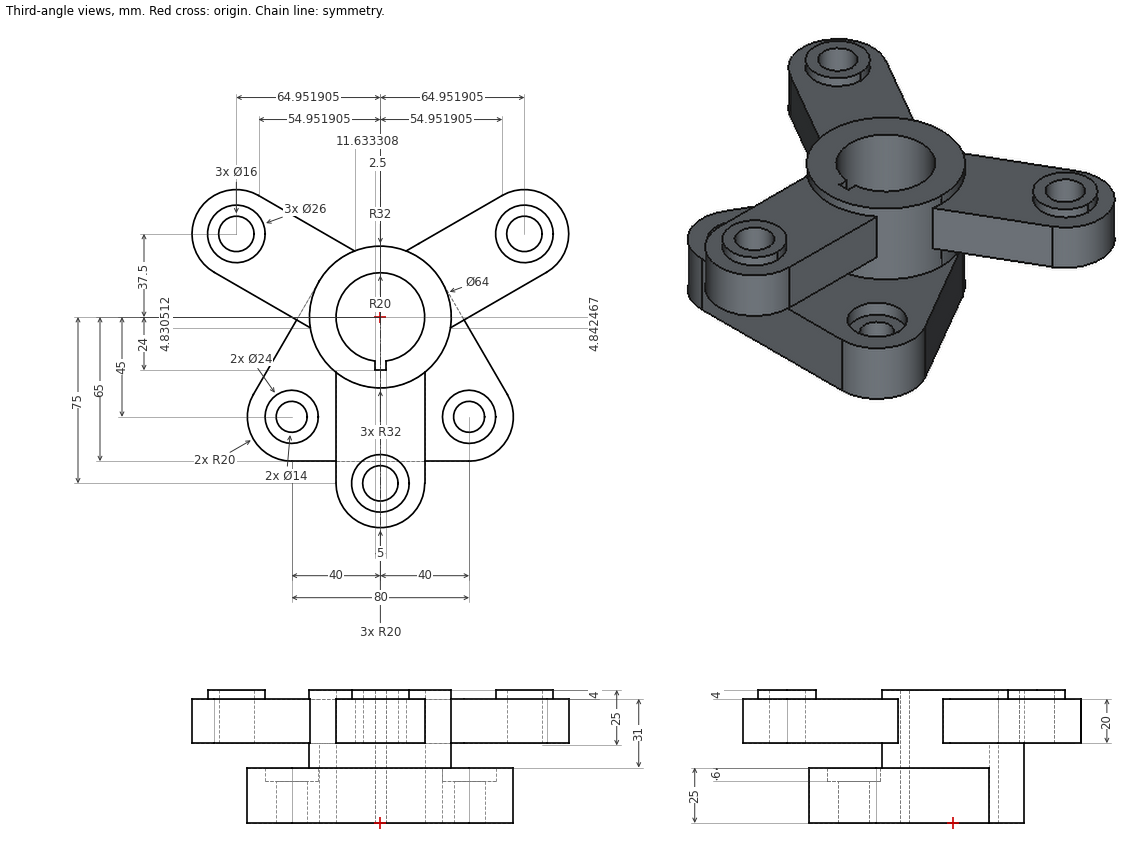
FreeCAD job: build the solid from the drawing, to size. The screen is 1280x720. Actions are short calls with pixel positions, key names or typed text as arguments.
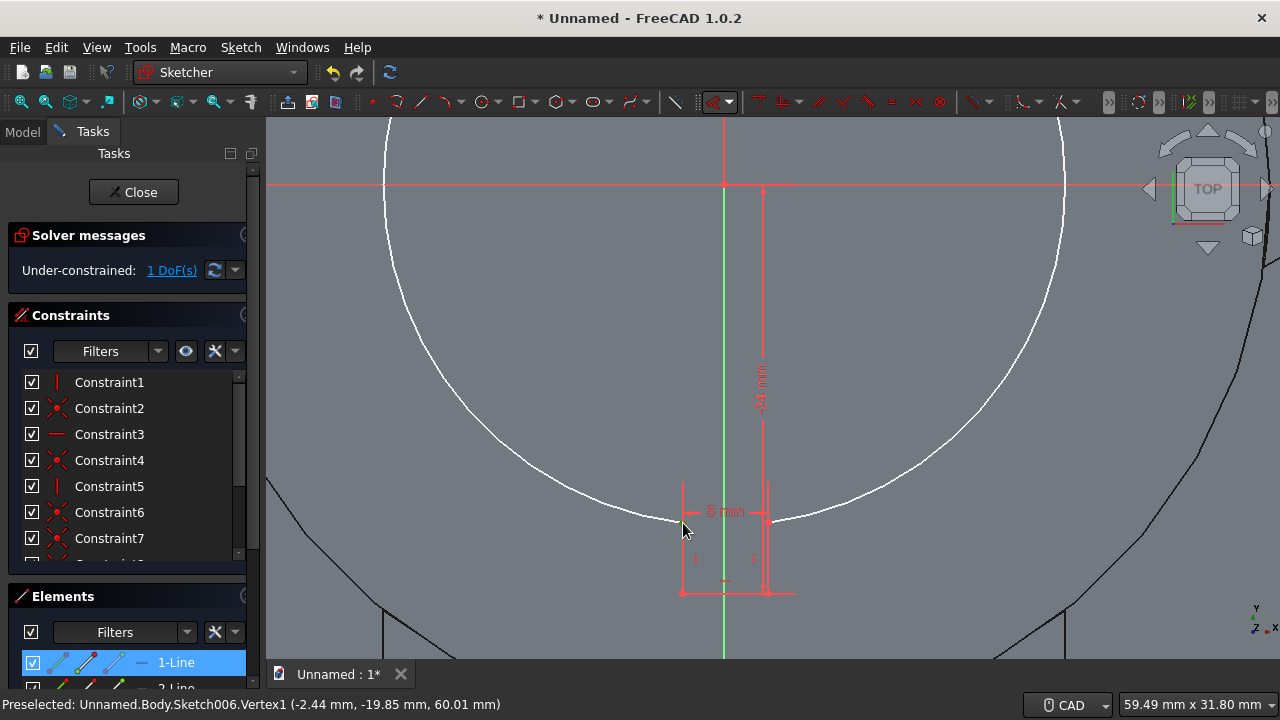
key(l)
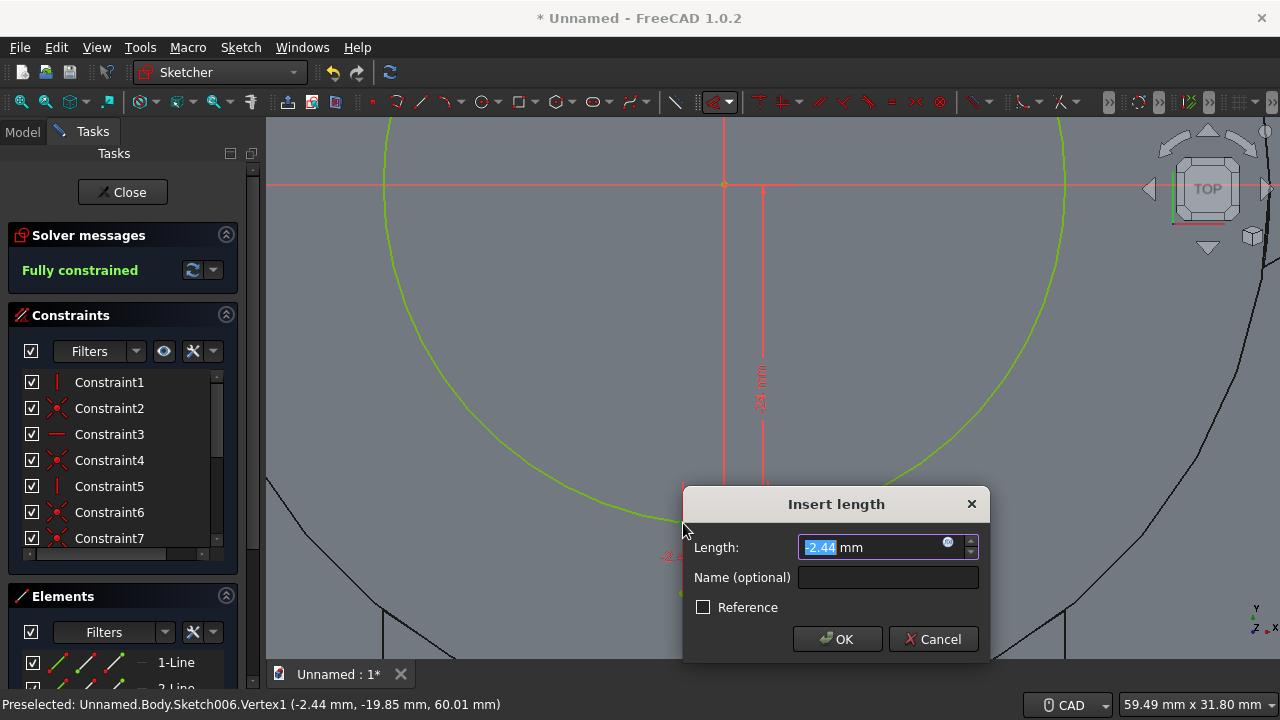
text(-2.5)
key(Return)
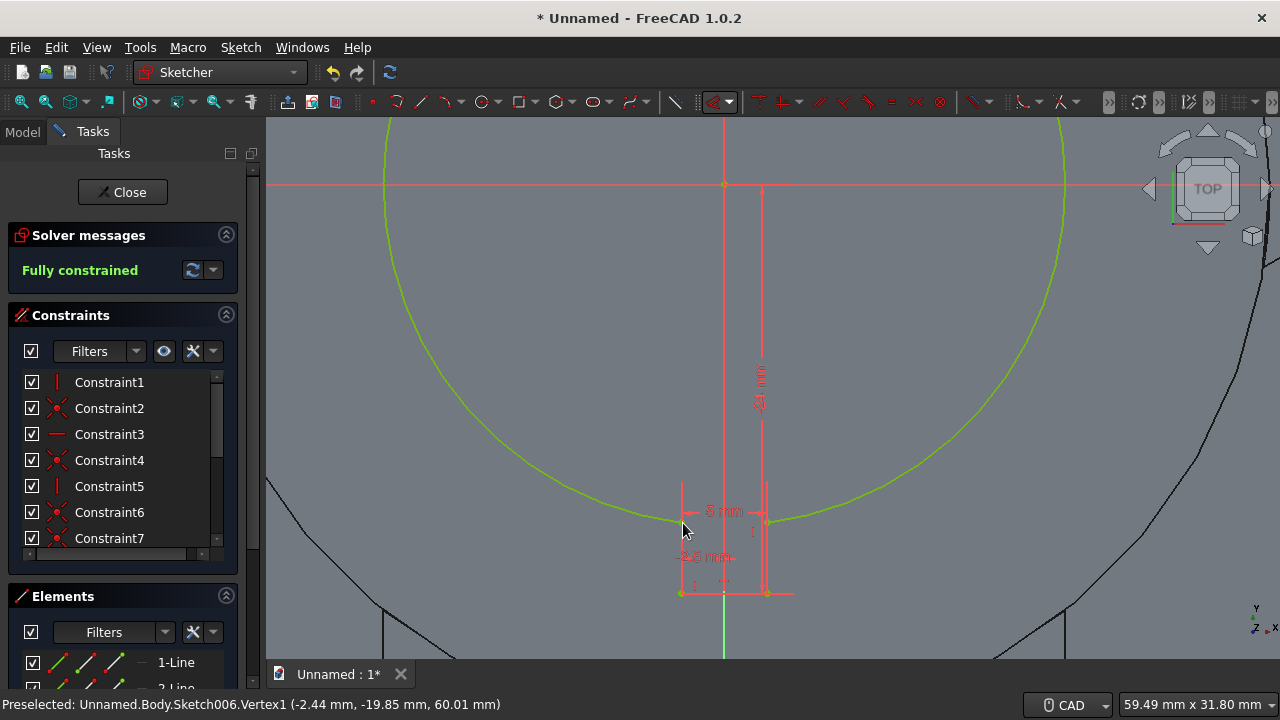
click(123, 192)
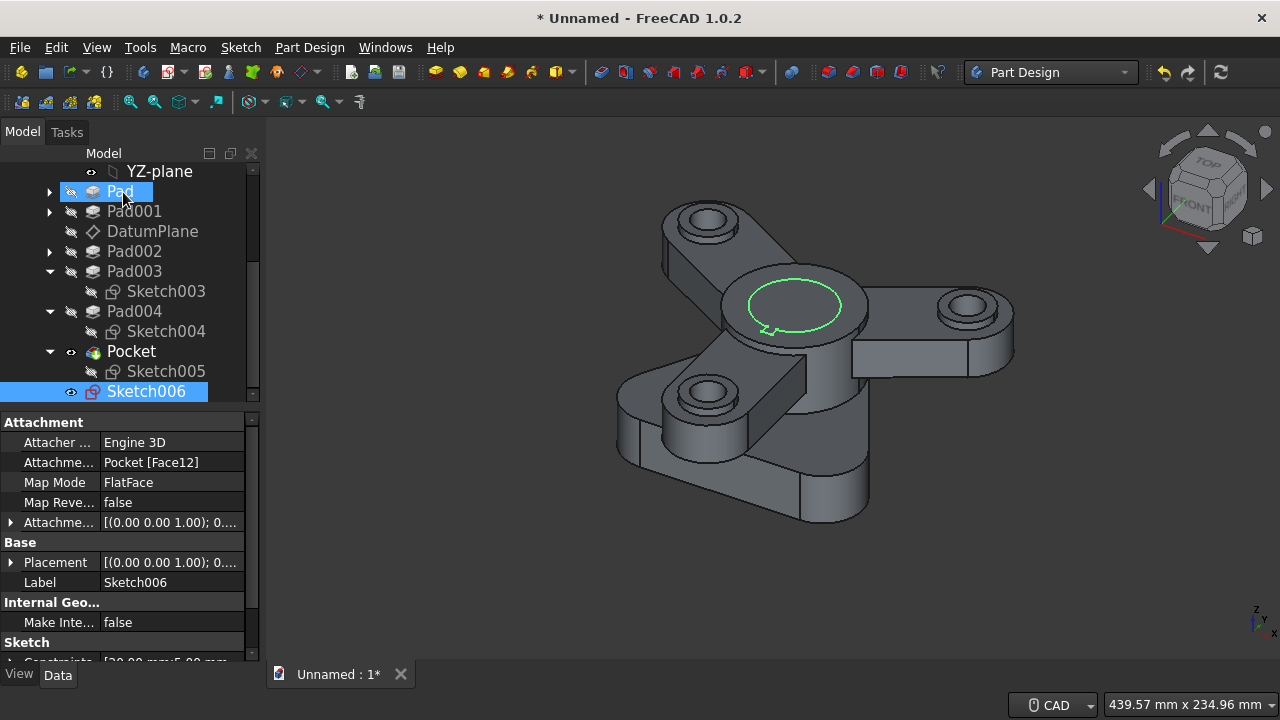
click(602, 72)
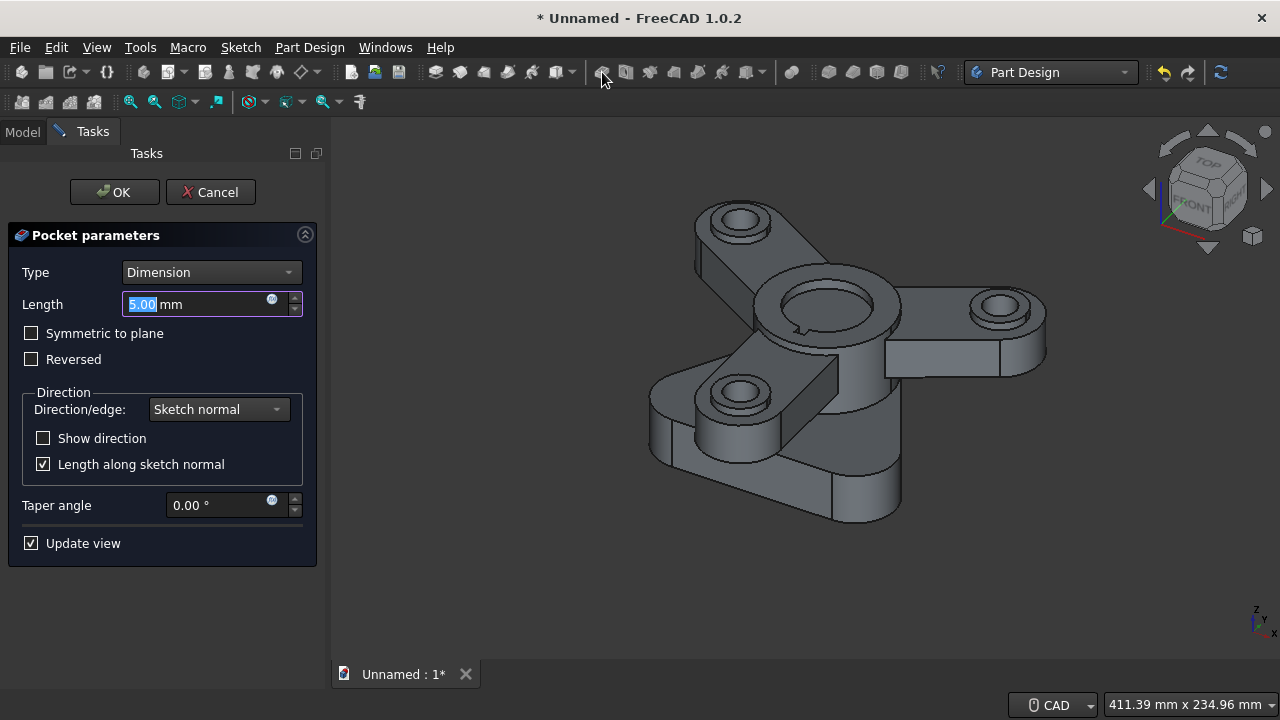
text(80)
key(Tab)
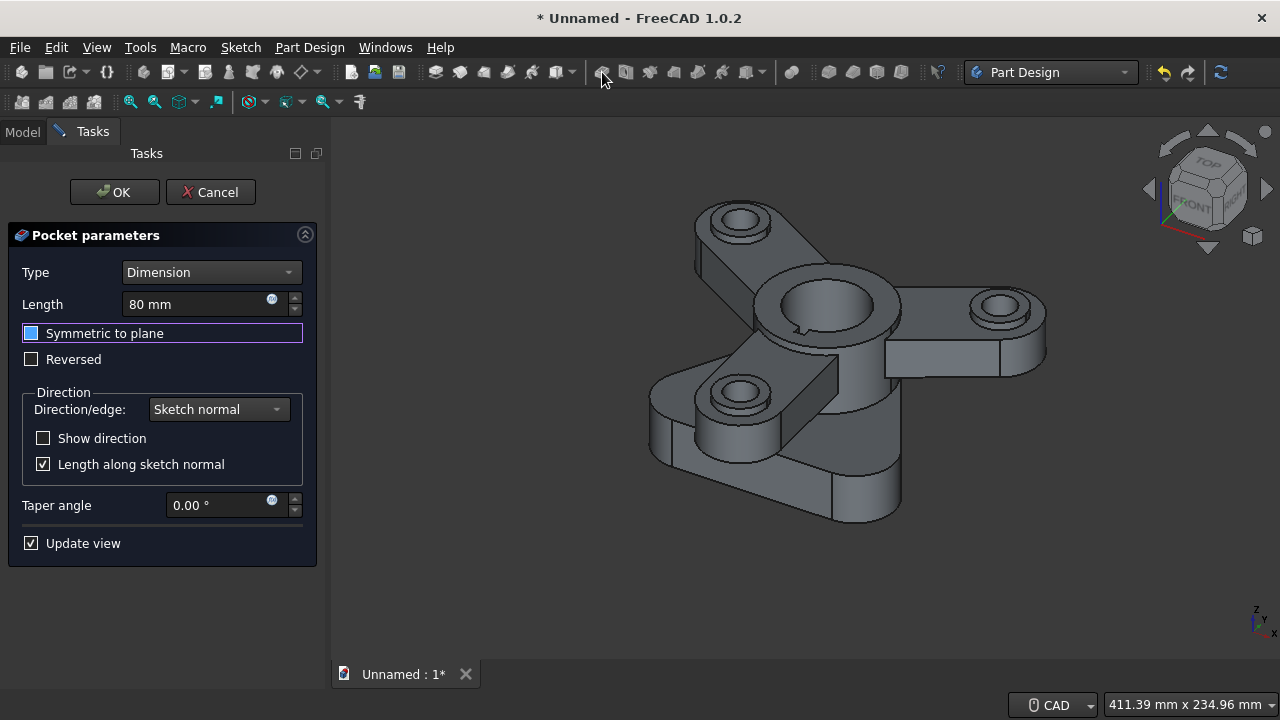
click(115, 192)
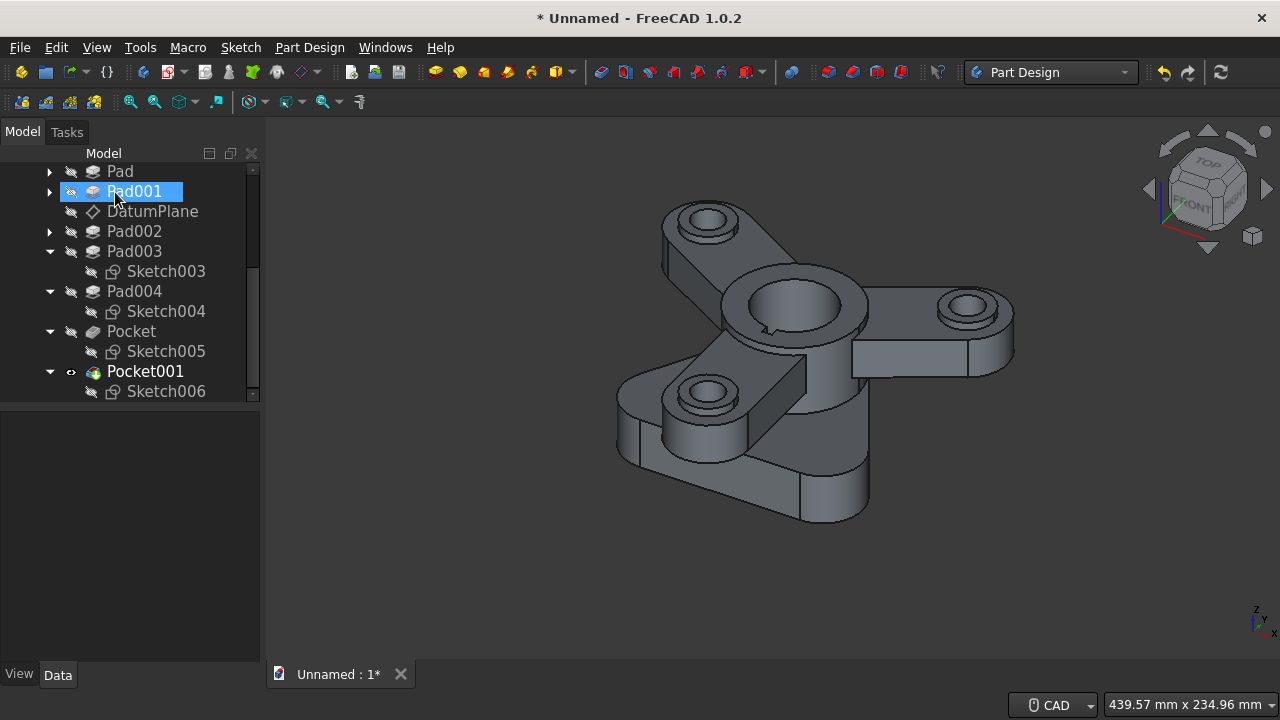
click(822, 435)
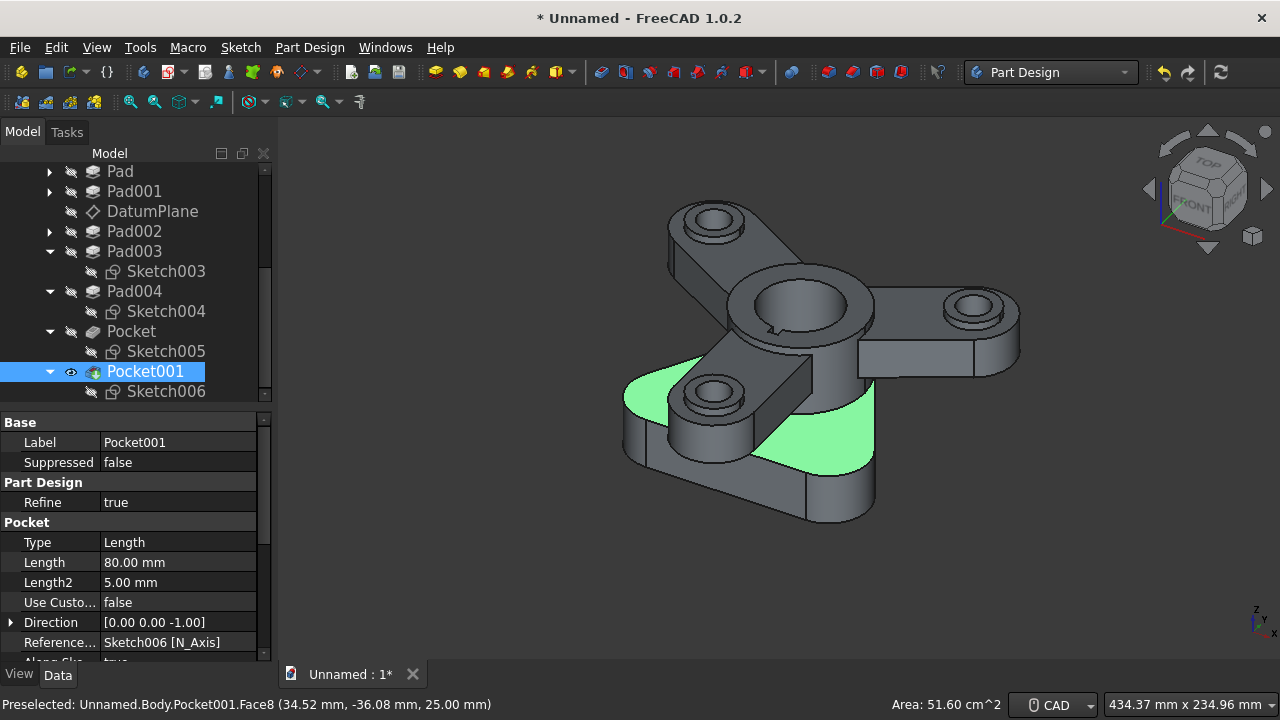
click(168, 72)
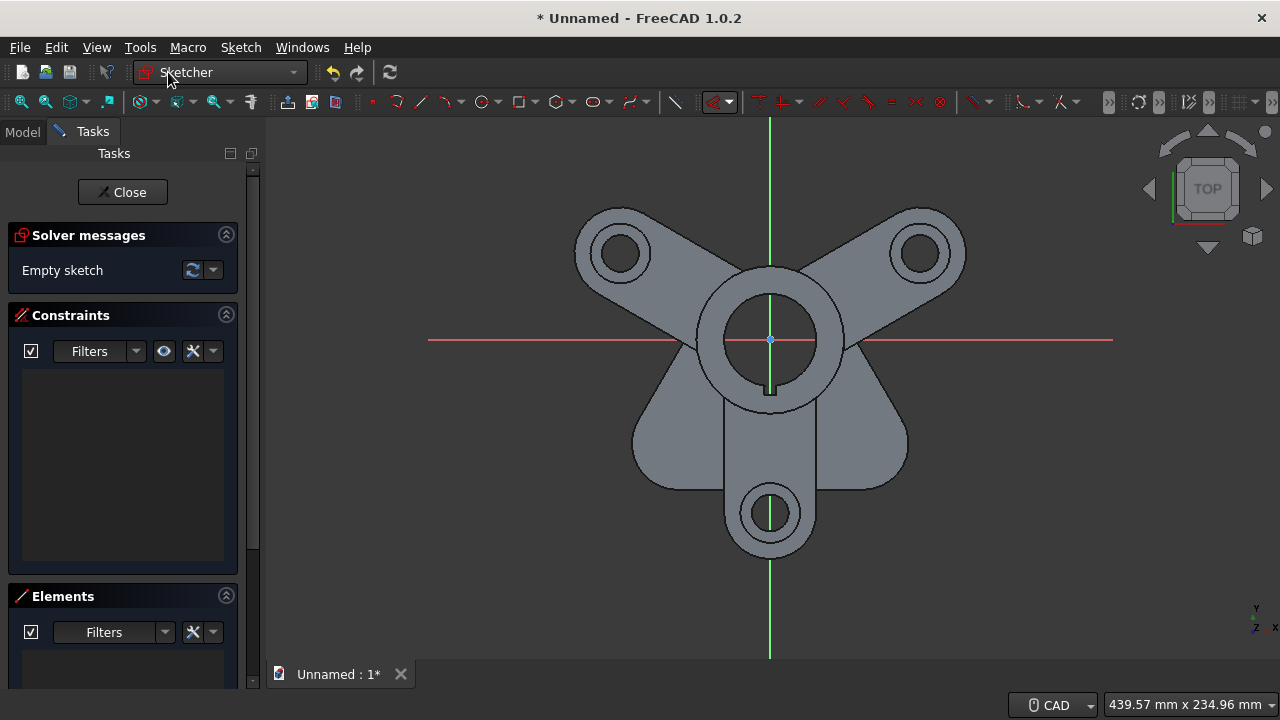
scroll(824, 420, up, 4)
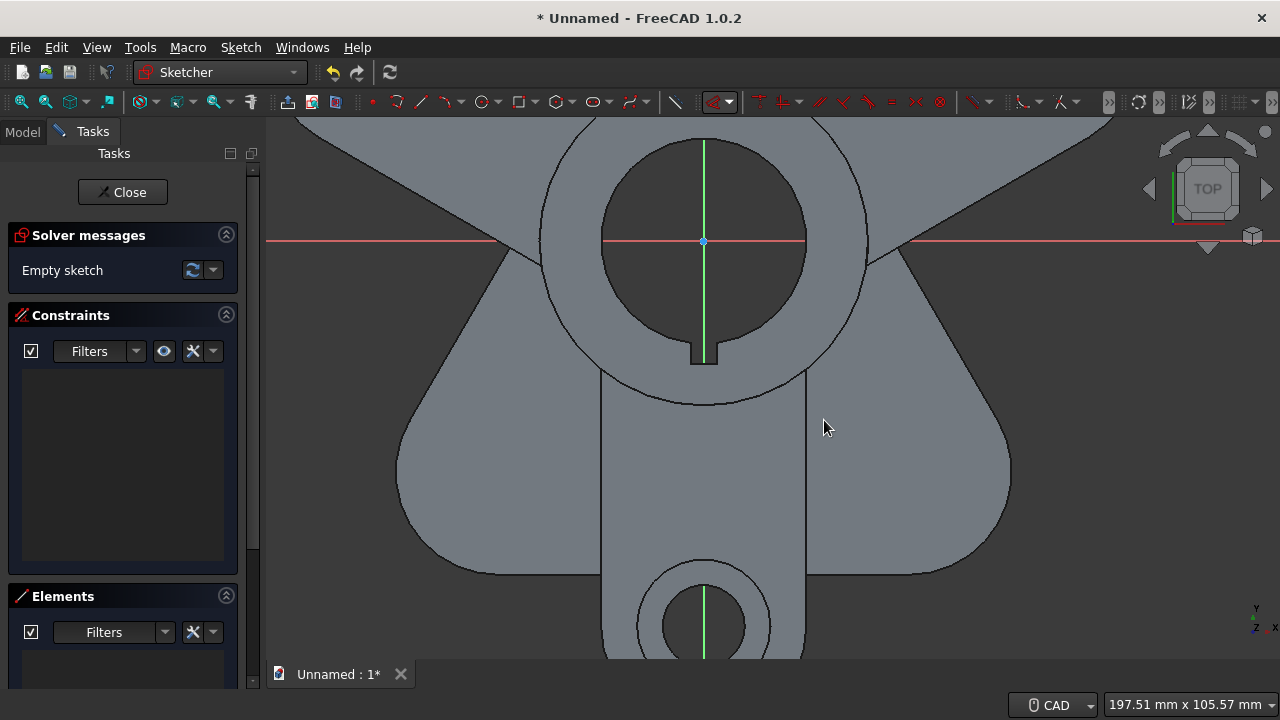
click(482, 102)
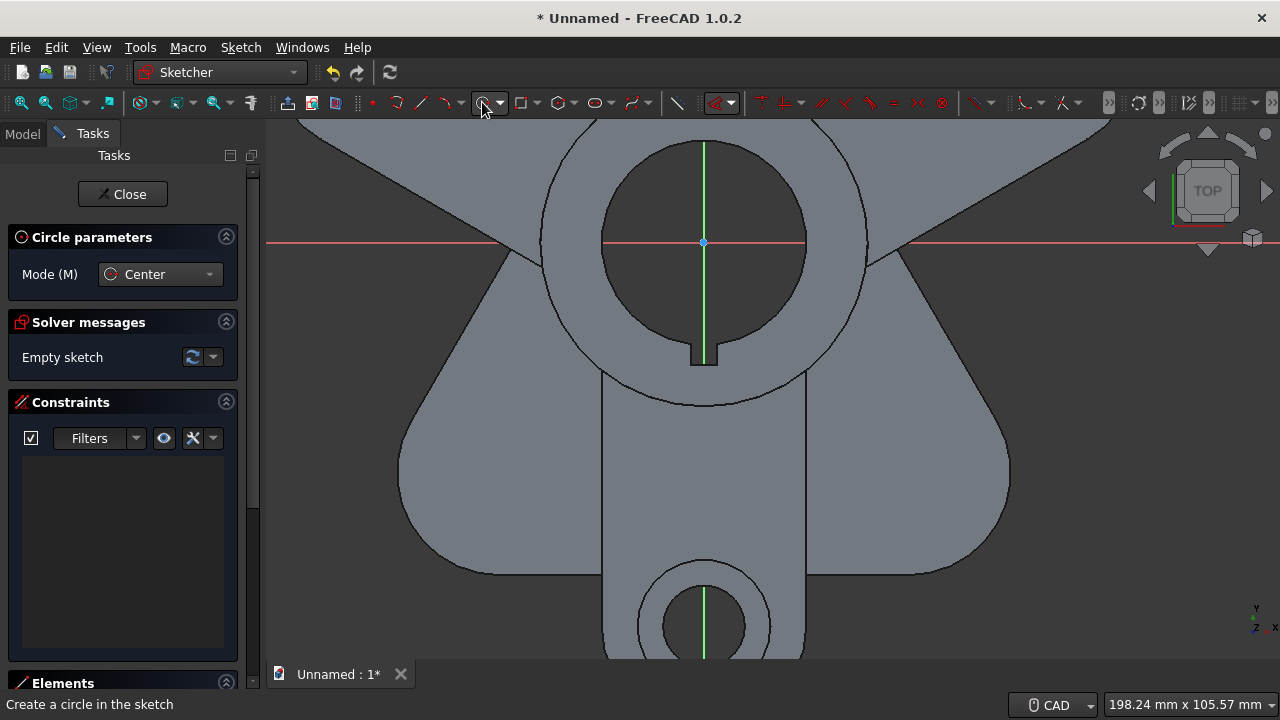
click(499, 473)
click(543, 429)